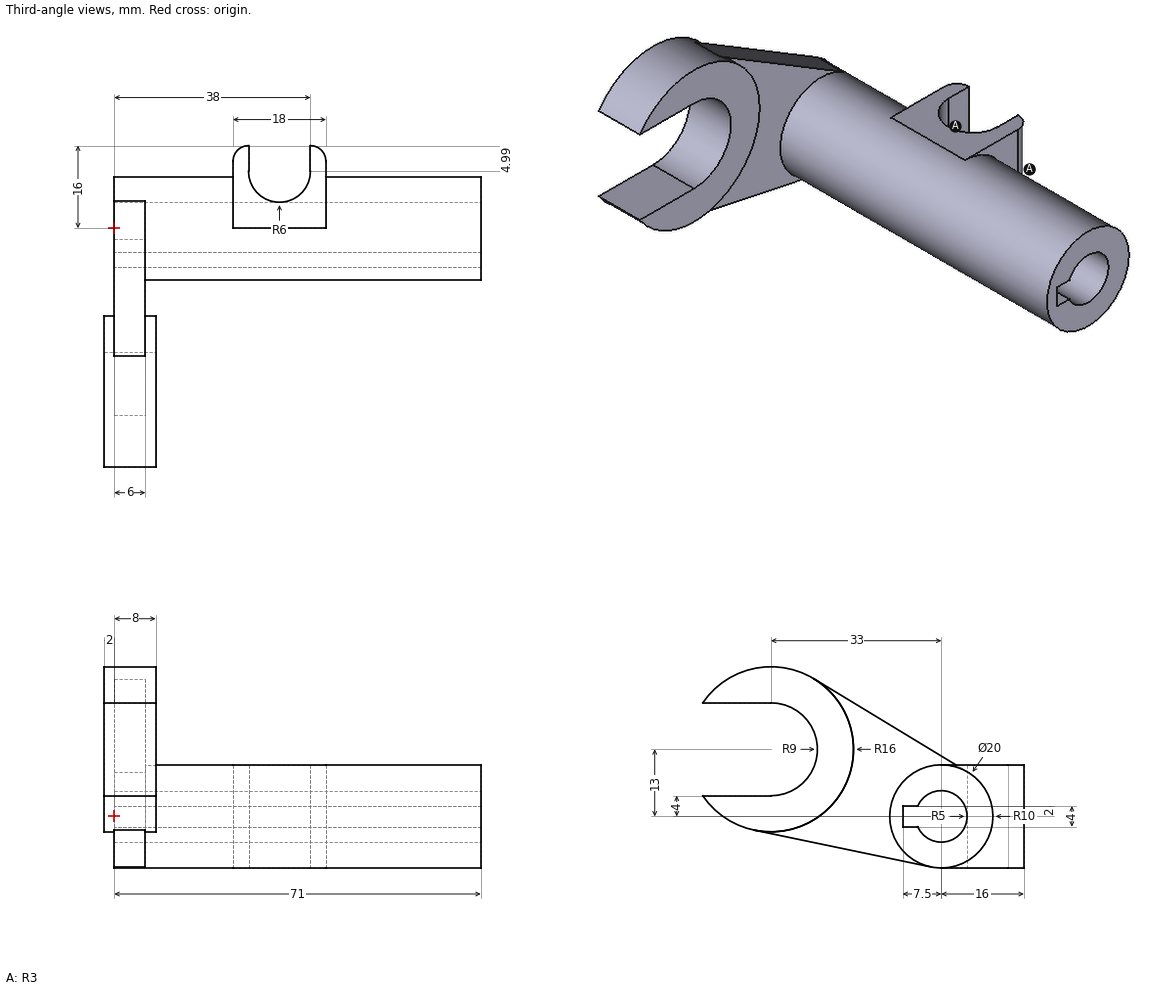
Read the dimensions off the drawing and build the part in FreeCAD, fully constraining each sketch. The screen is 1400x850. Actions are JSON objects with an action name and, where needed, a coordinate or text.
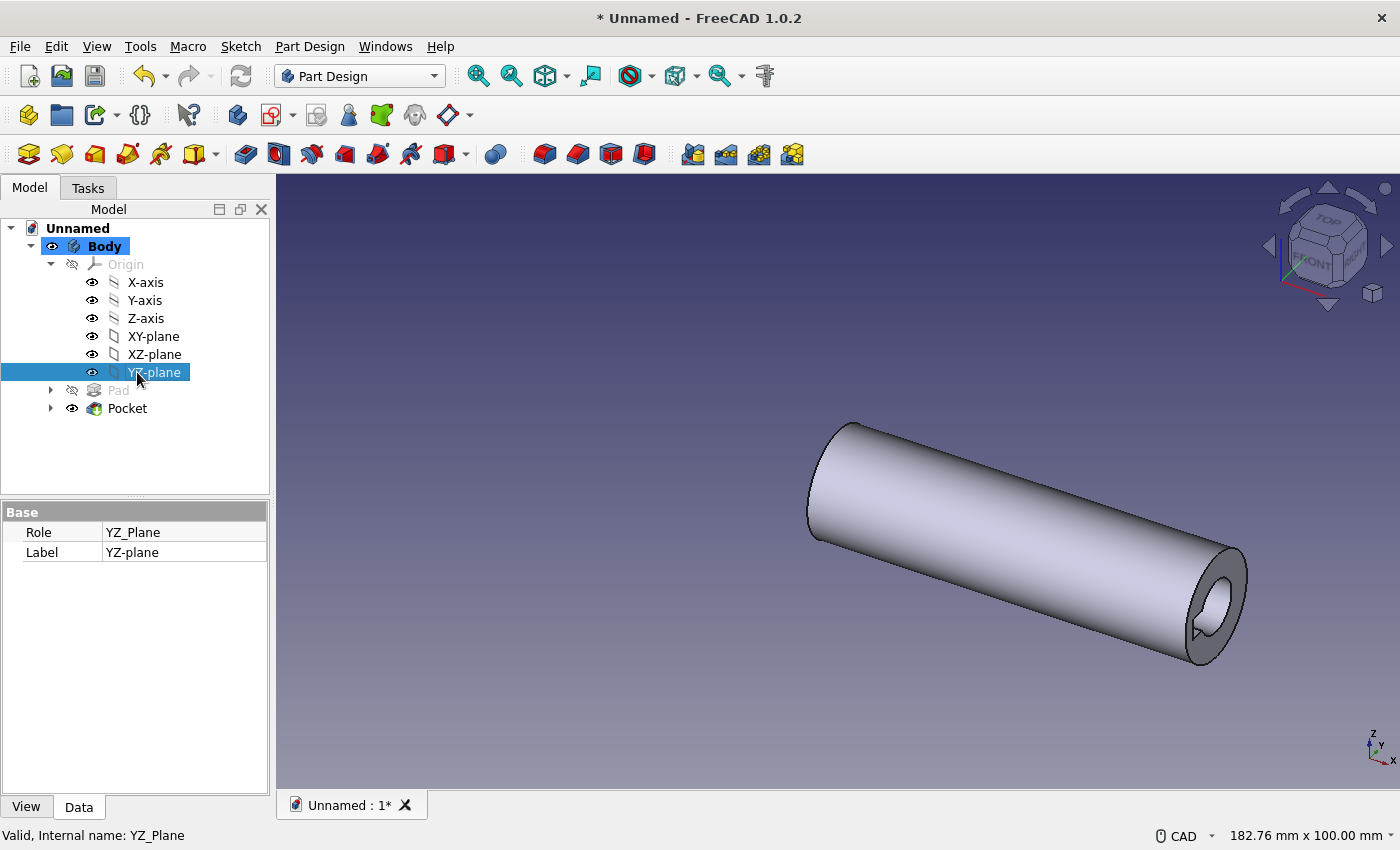
{"action": "left_click", "coordinate": [448, 116]}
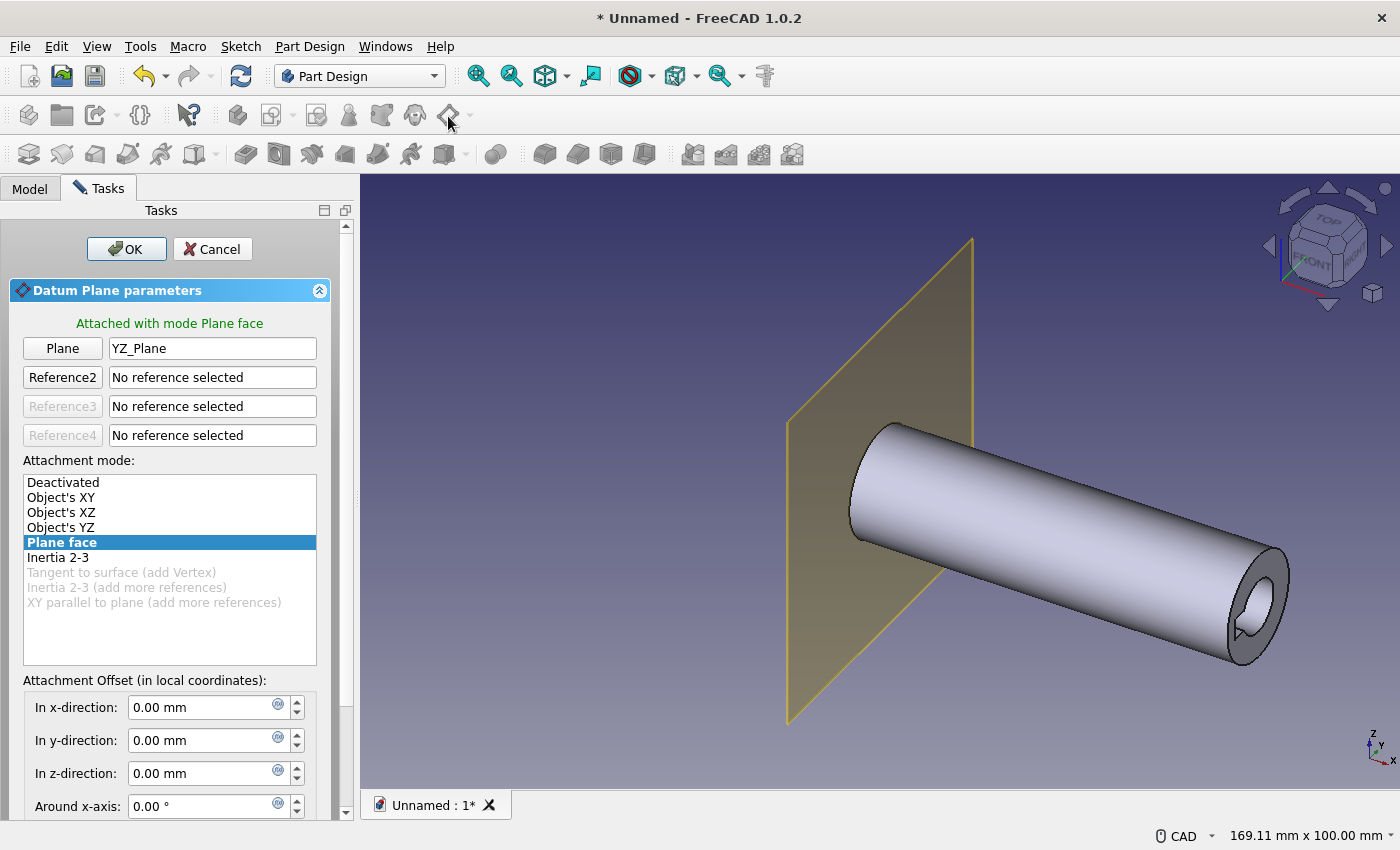
{"action": "triple_click", "coordinate": [210, 774]}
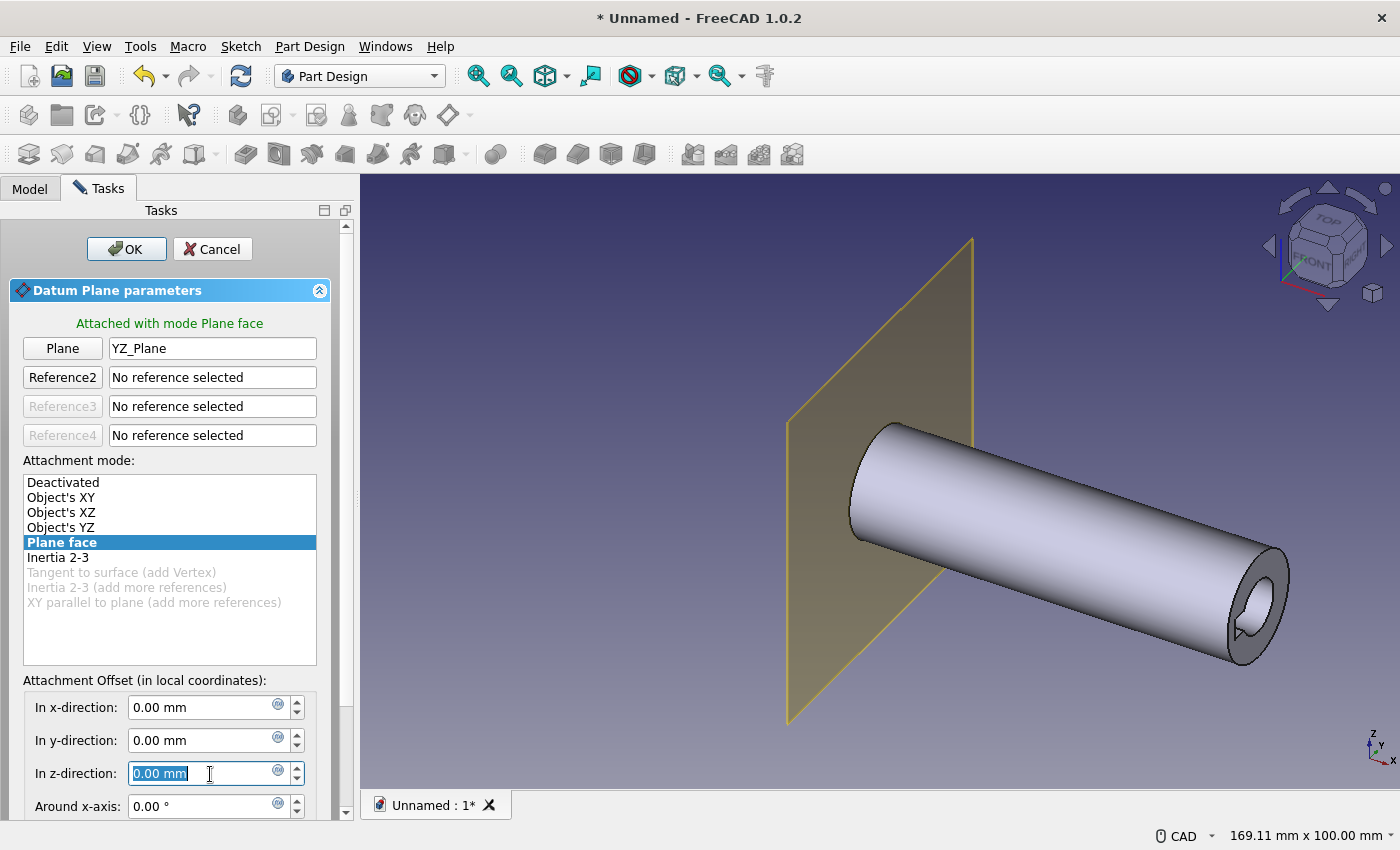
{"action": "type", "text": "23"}
{"action": "key", "text": "Tab"}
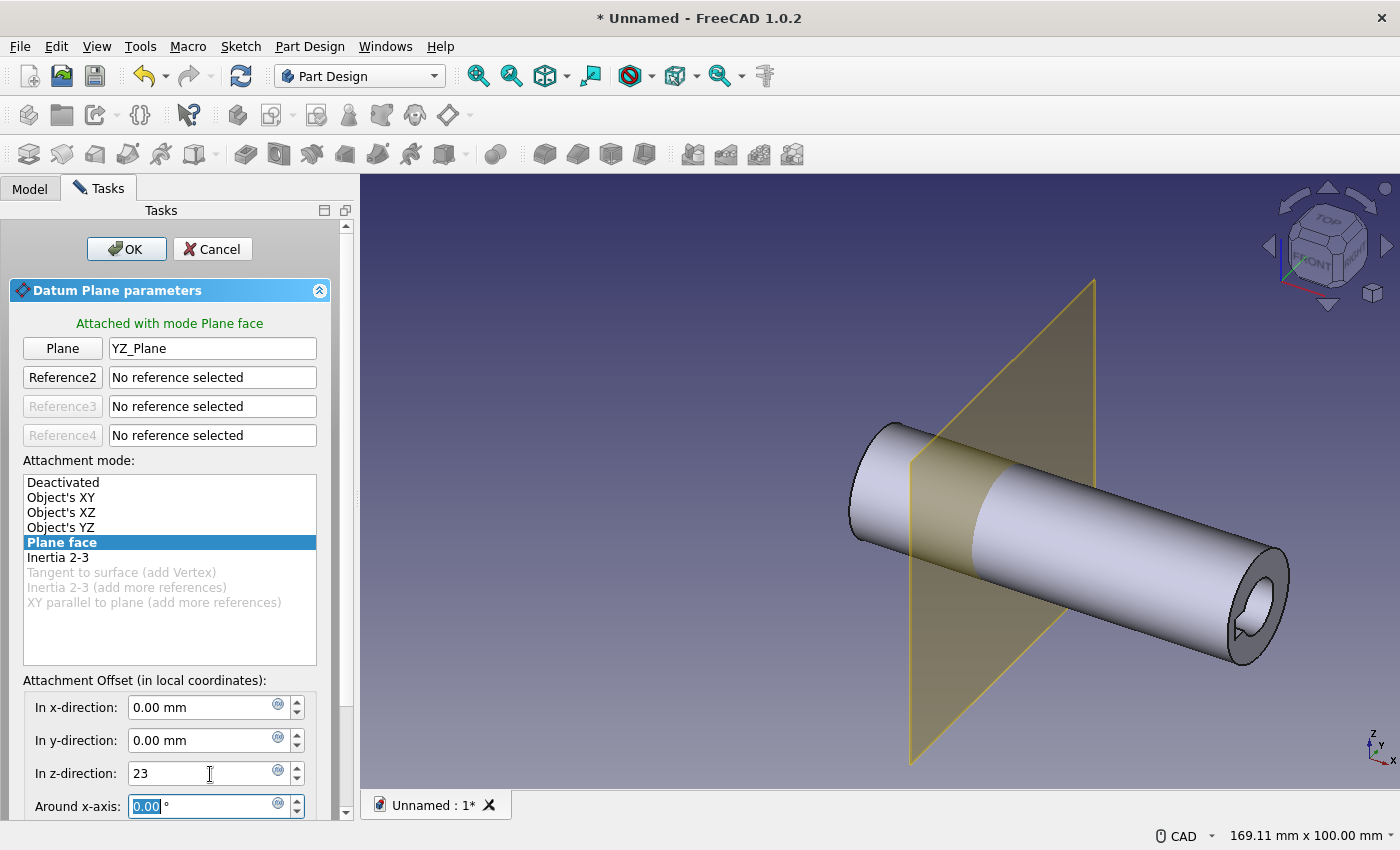
{"action": "left_click", "coordinate": [127, 249]}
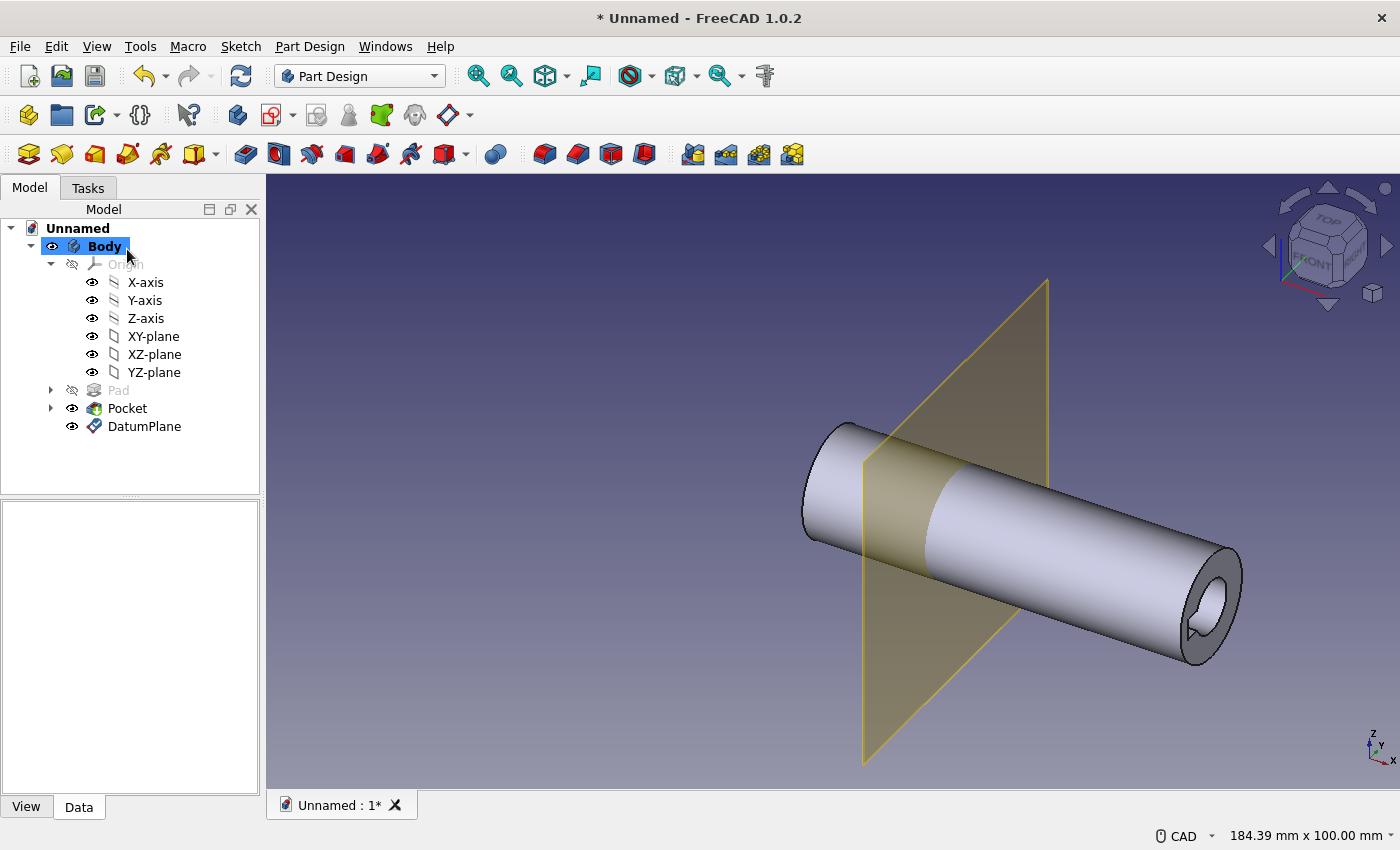
{"action": "left_click", "coordinate": [117, 426]}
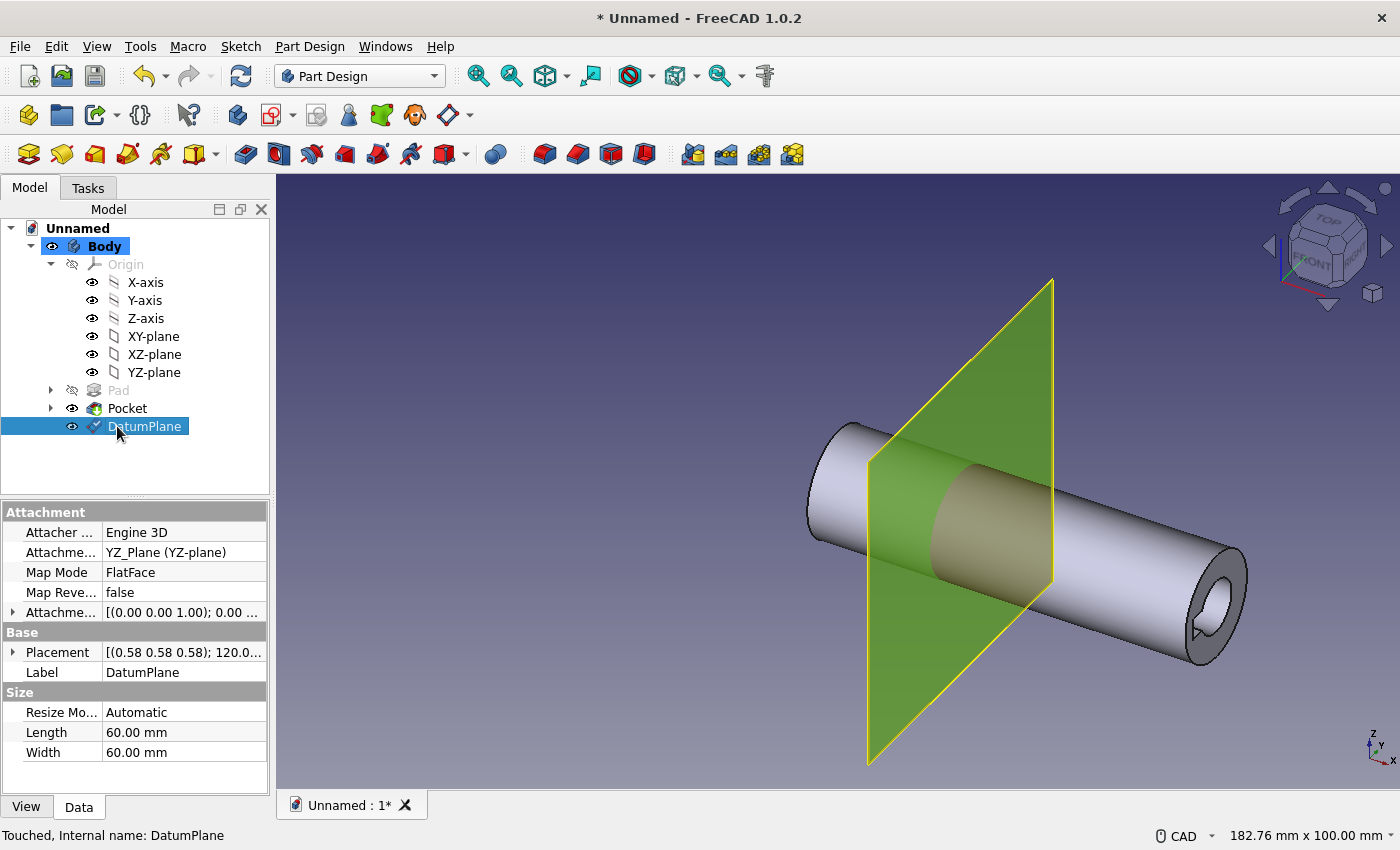
{"action": "left_click", "coordinate": [270, 116]}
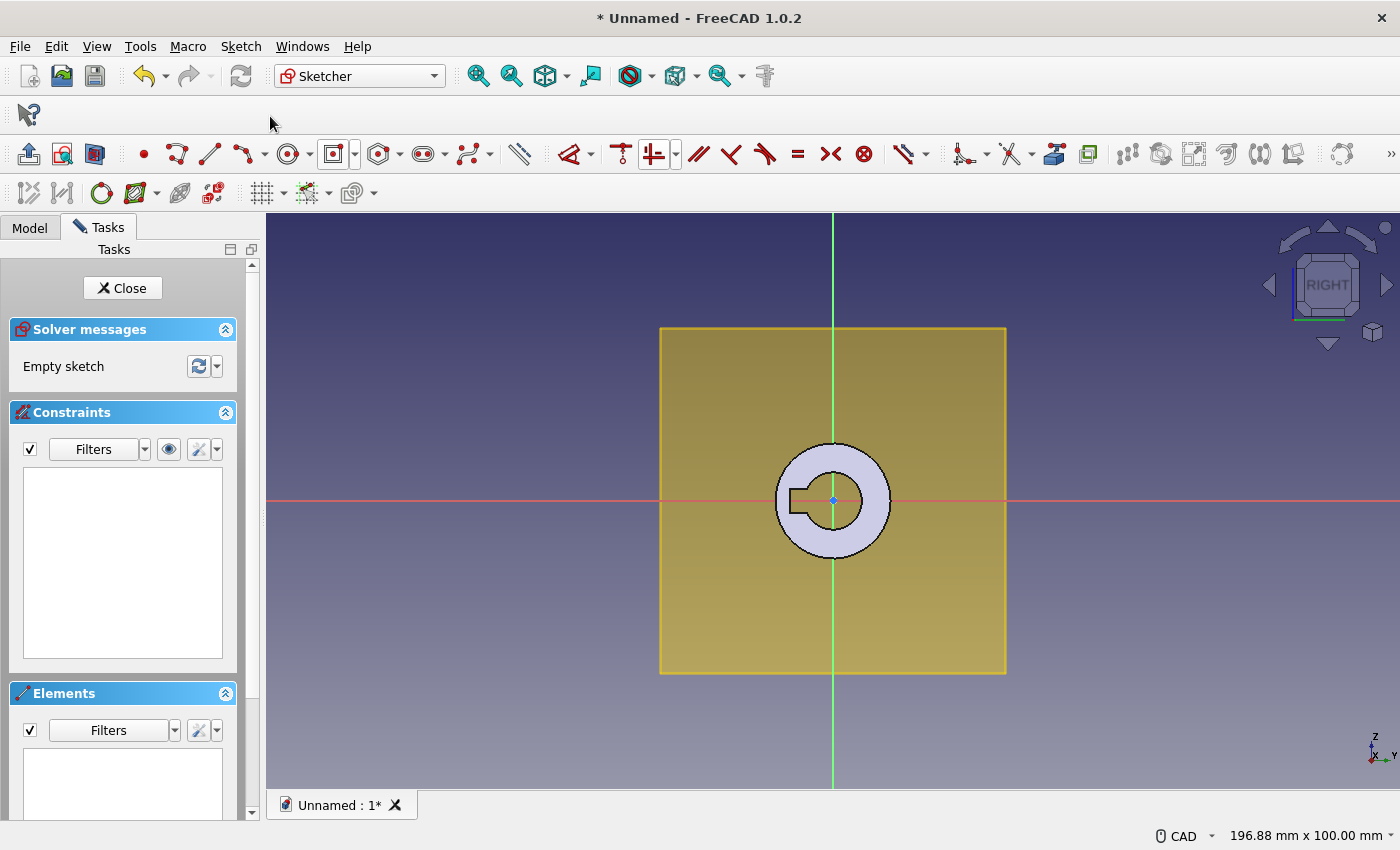
{"action": "key", "text": "q s"}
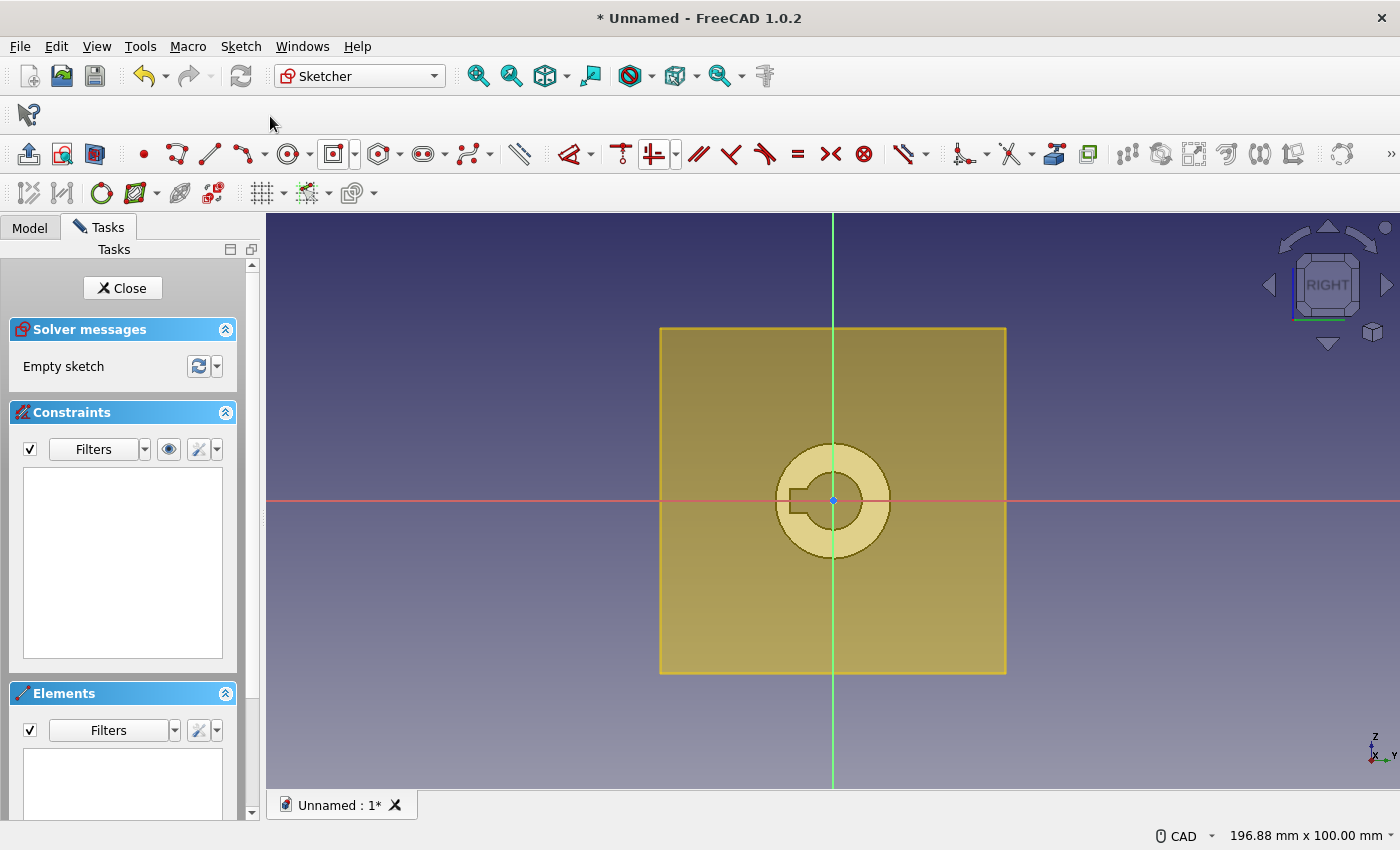
{"action": "scroll", "coordinate": [928, 501], "scroll_direction": "up", "scroll_amount": 6}